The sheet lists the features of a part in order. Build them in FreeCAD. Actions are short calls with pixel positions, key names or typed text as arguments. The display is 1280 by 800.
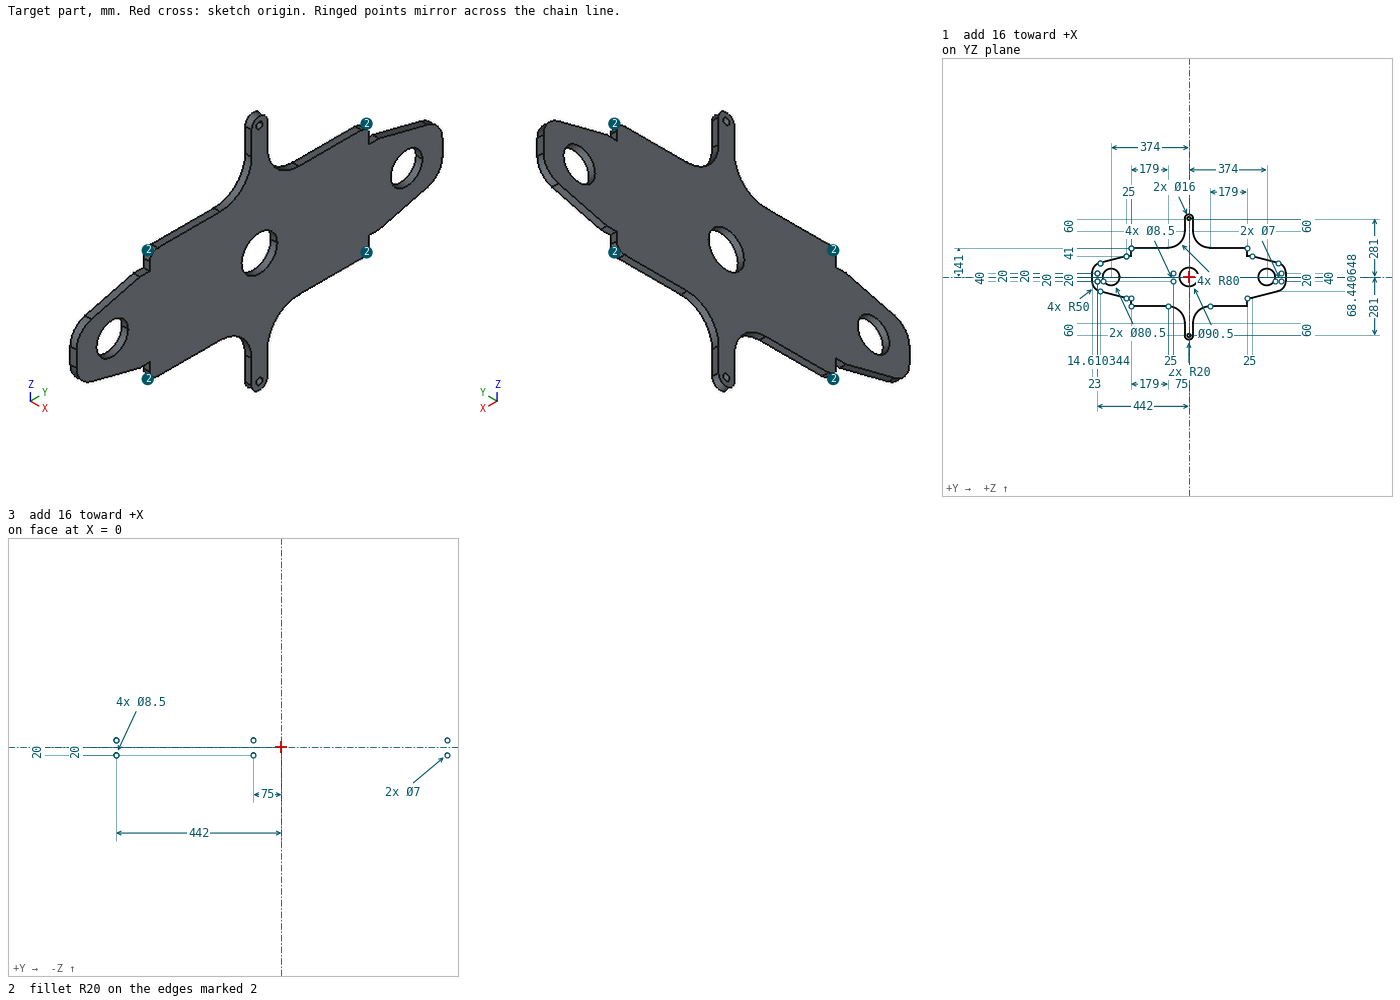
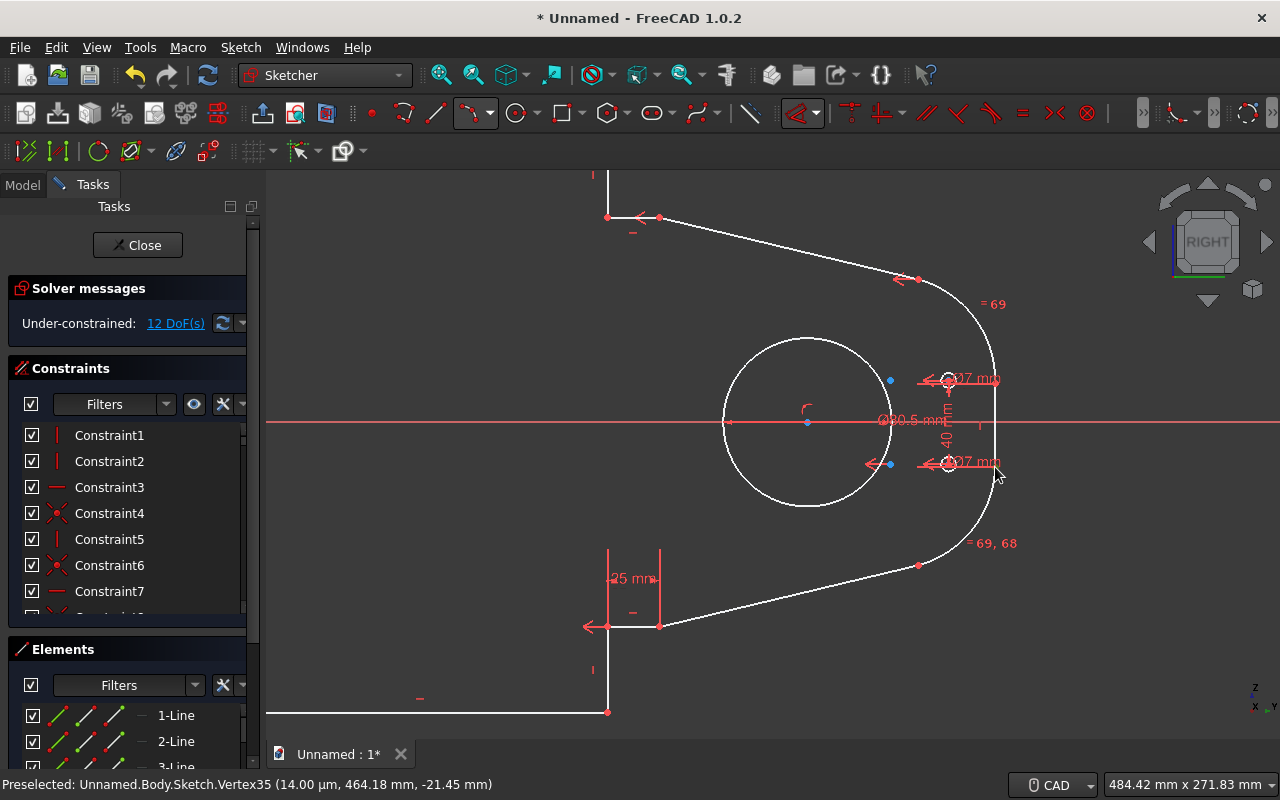
key(i)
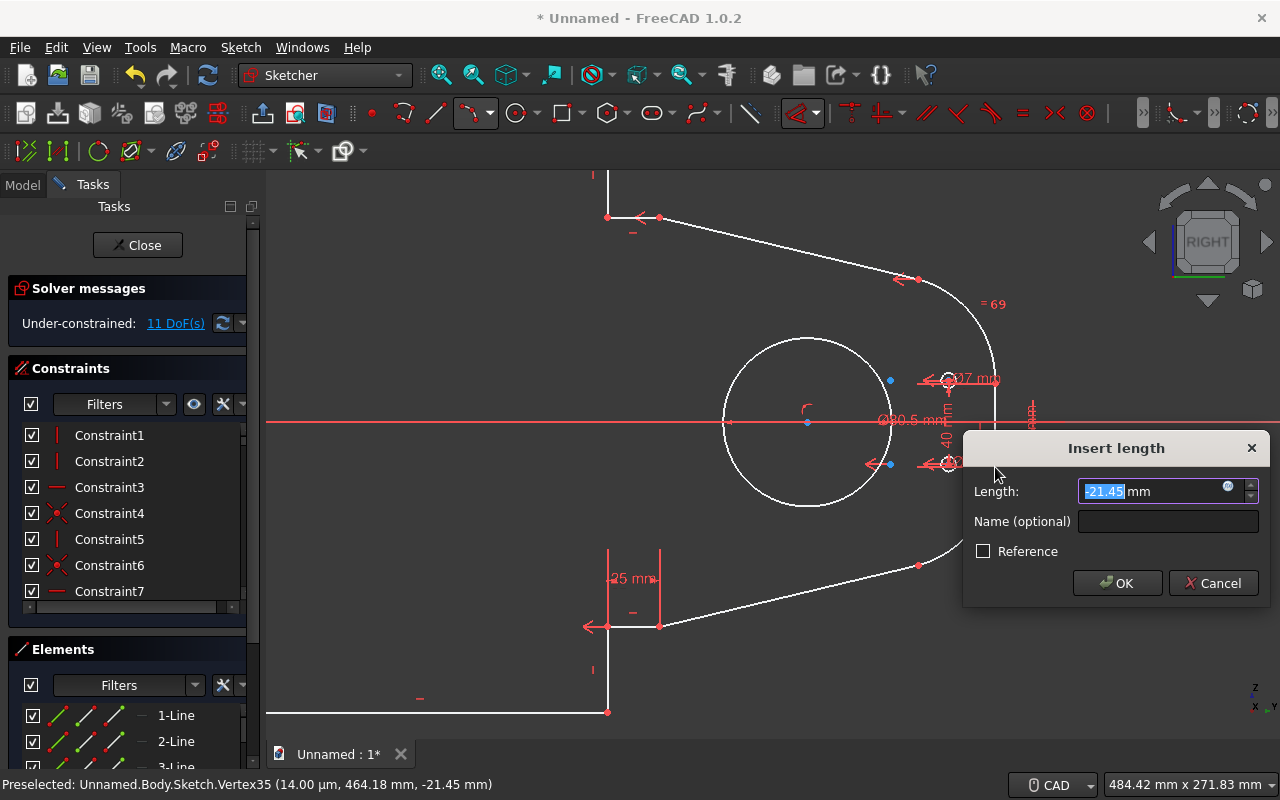
text(-20)
key(Return)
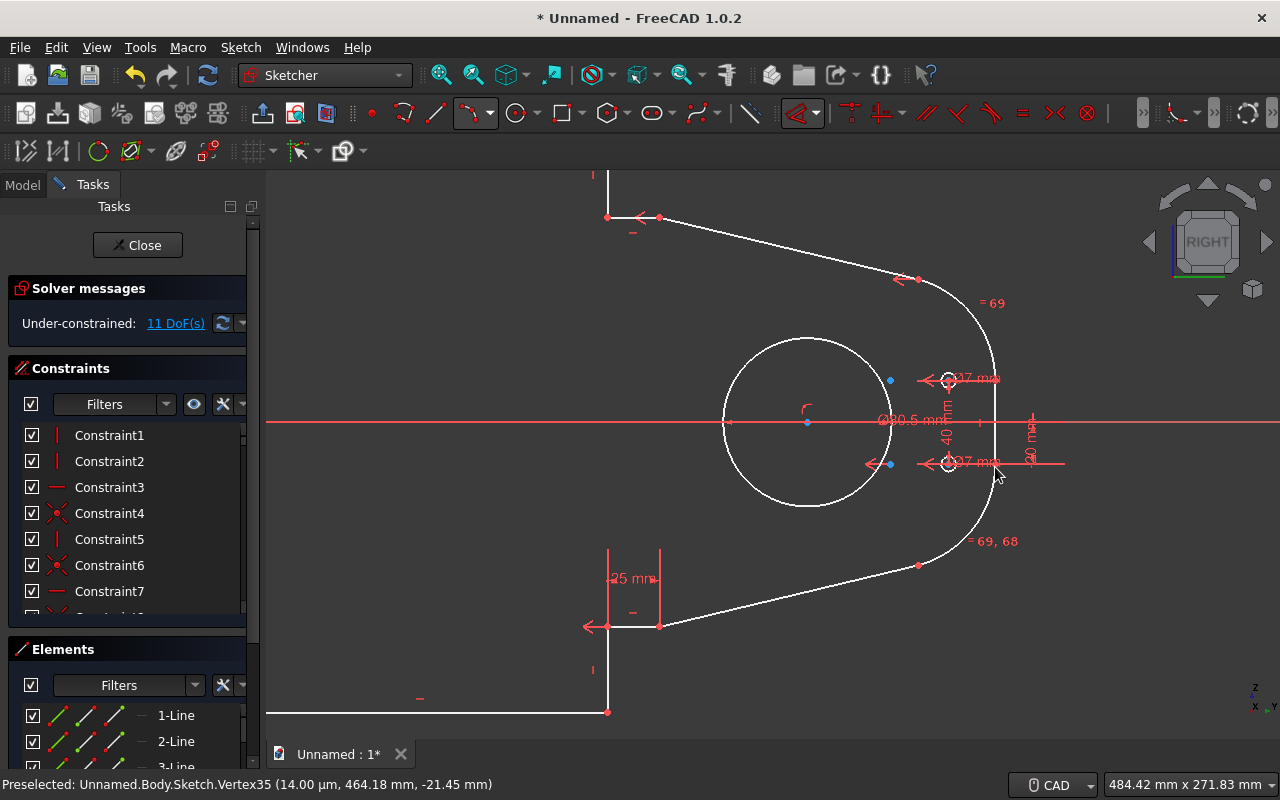
scroll(998, 468, down, 6)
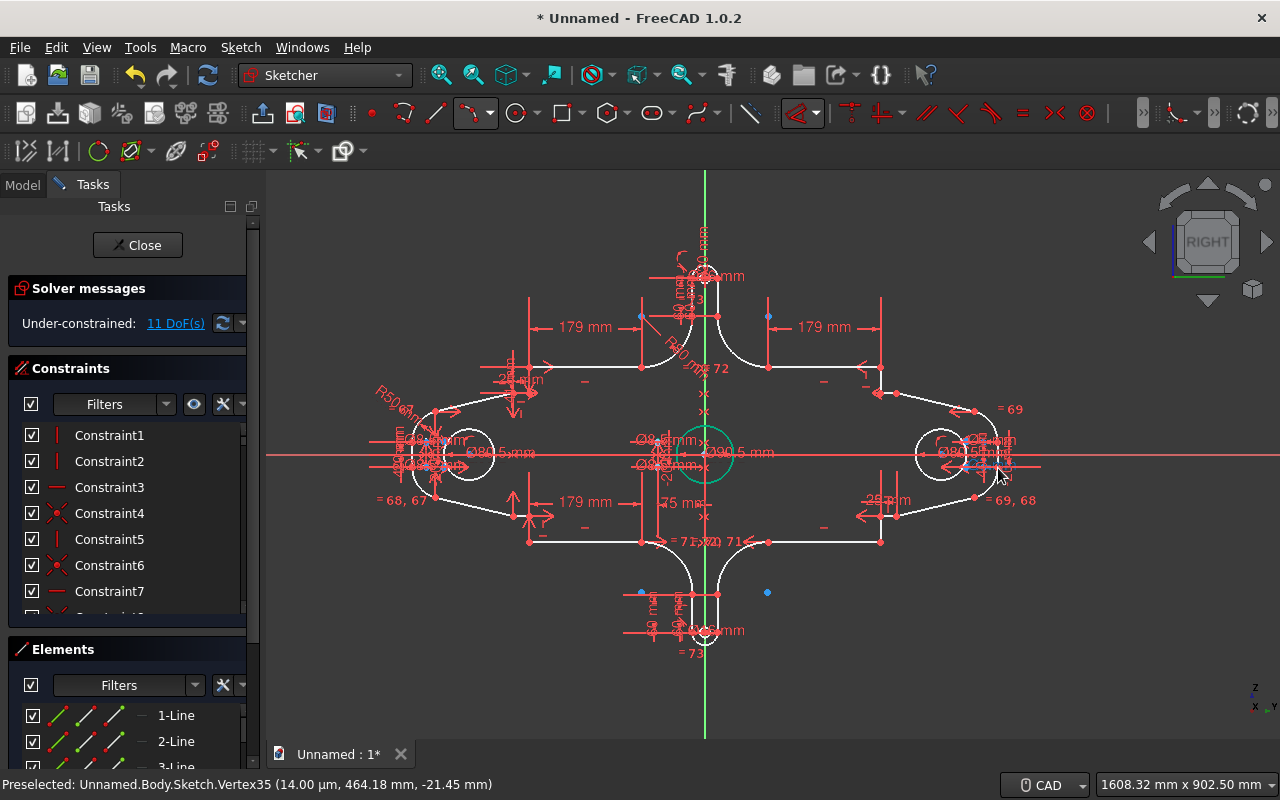
scroll(444, 442, up, 6)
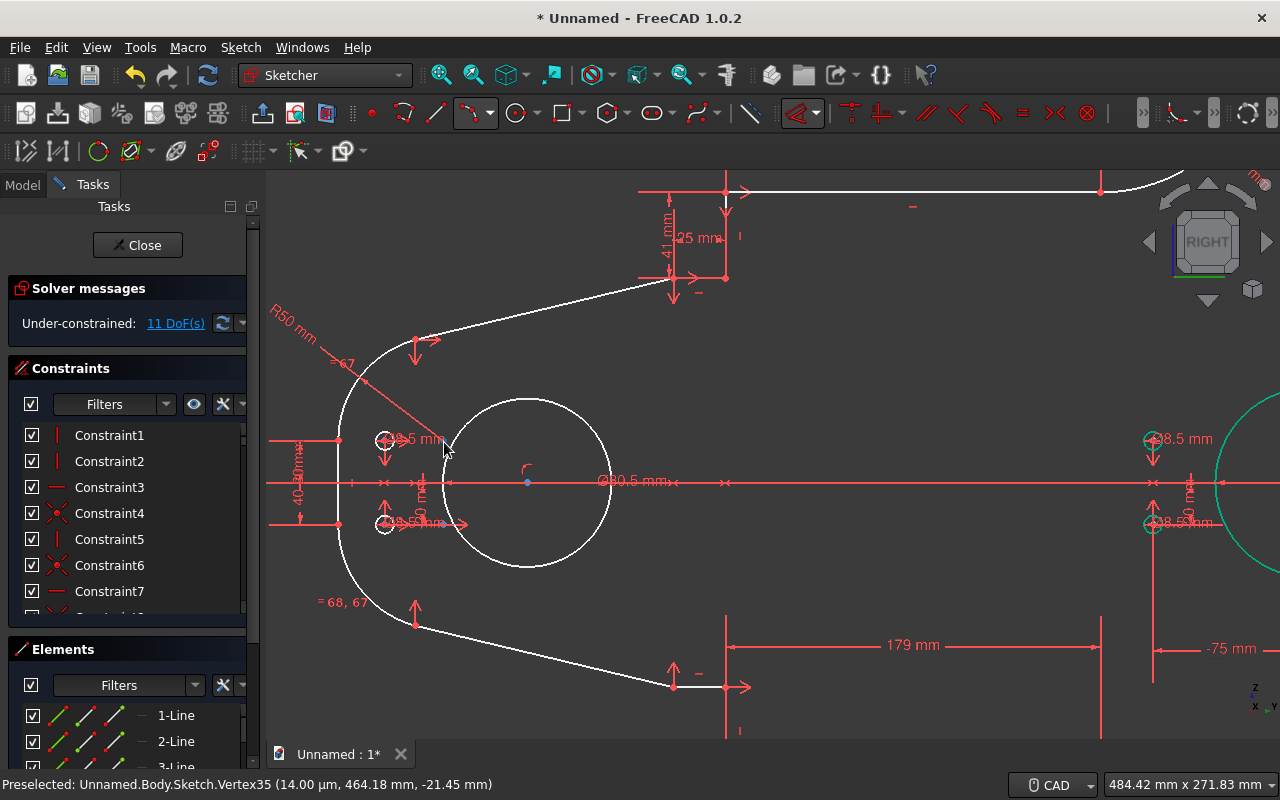
click(443, 441)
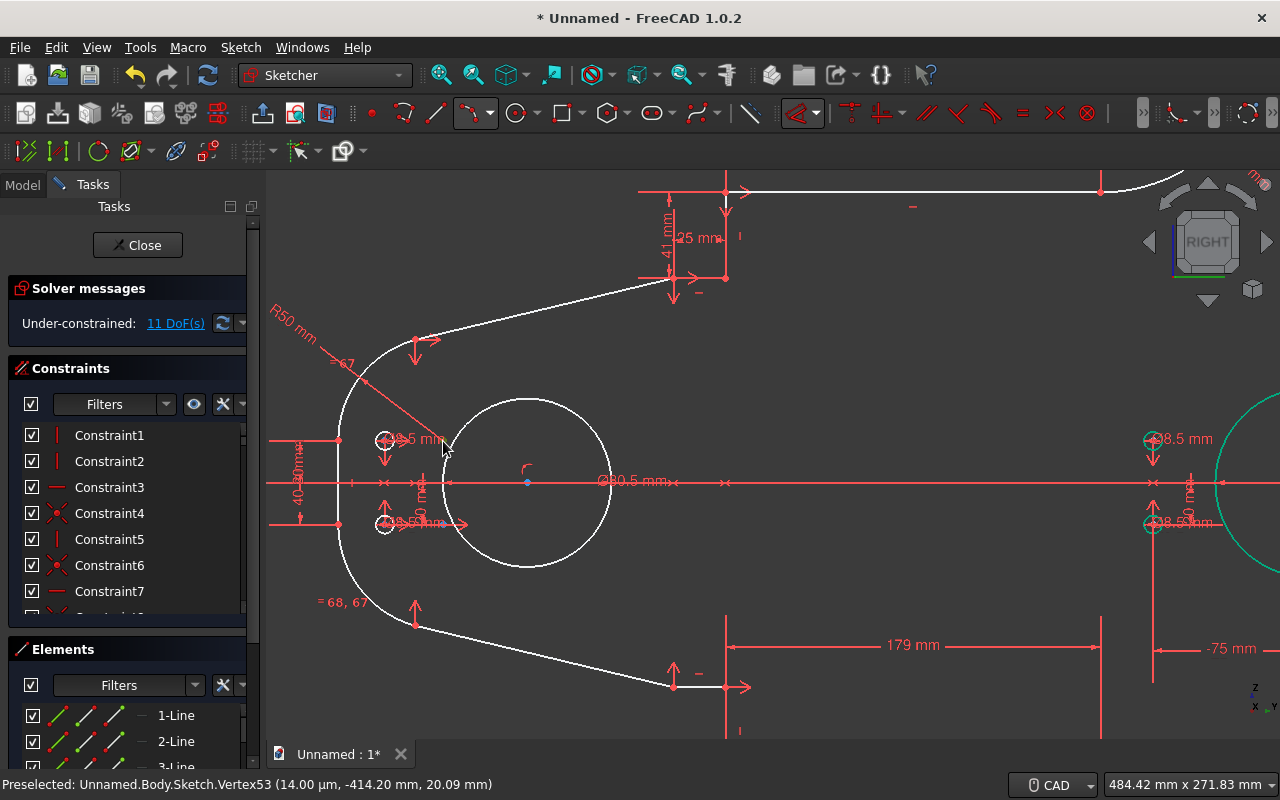
click(818, 114)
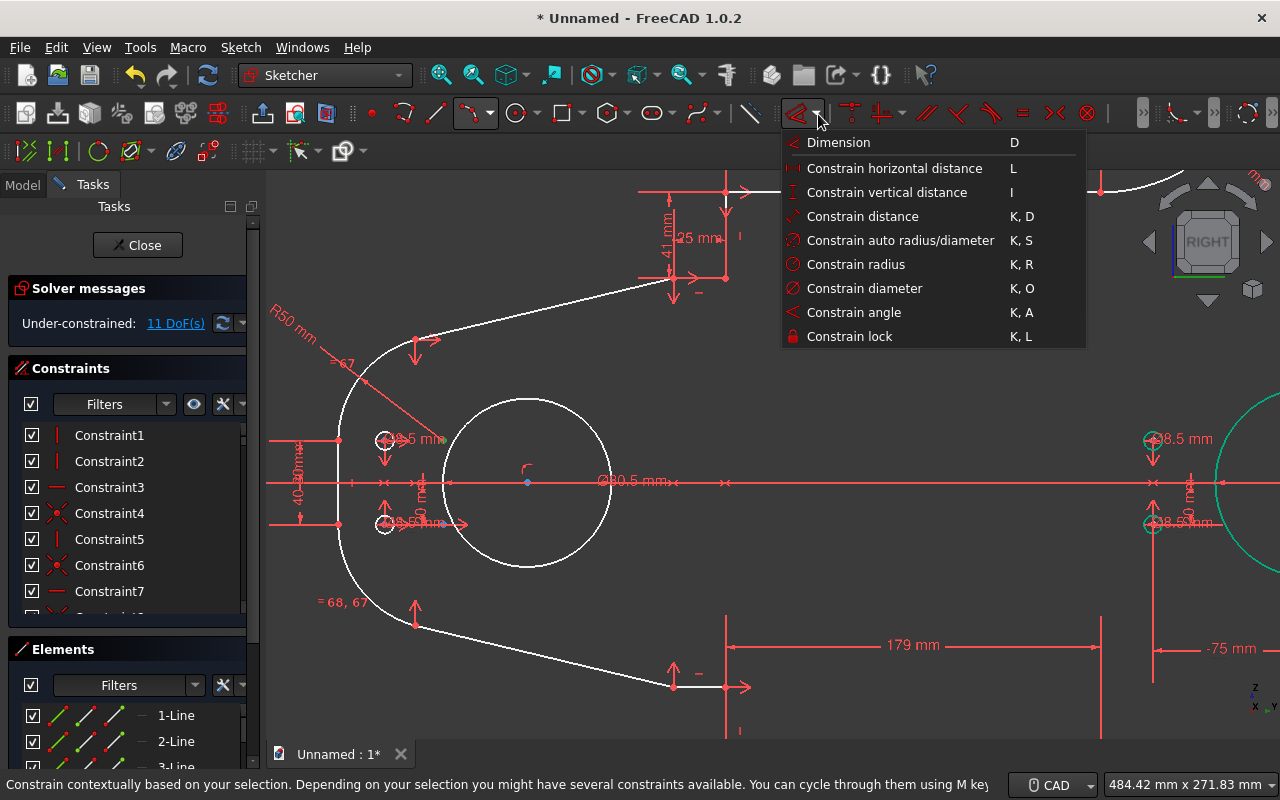
click(934, 192)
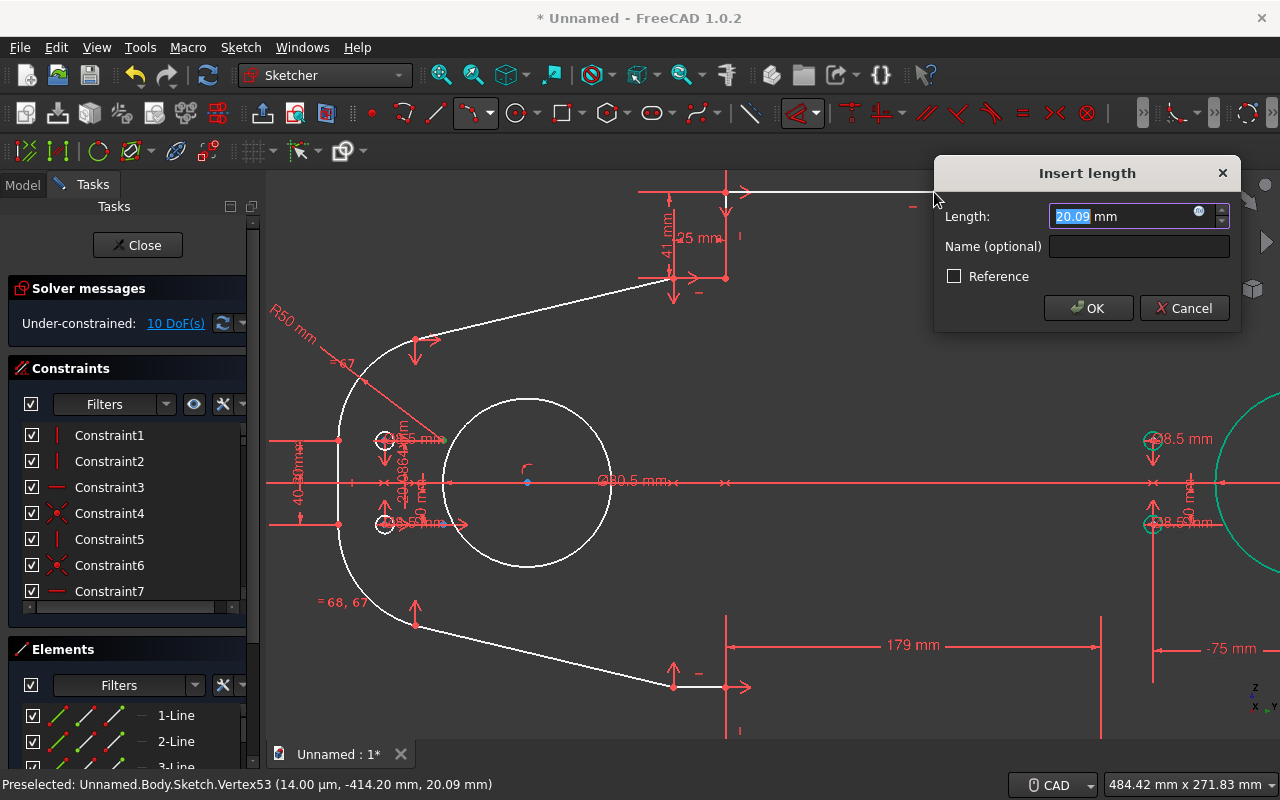
text(20)
key(Return)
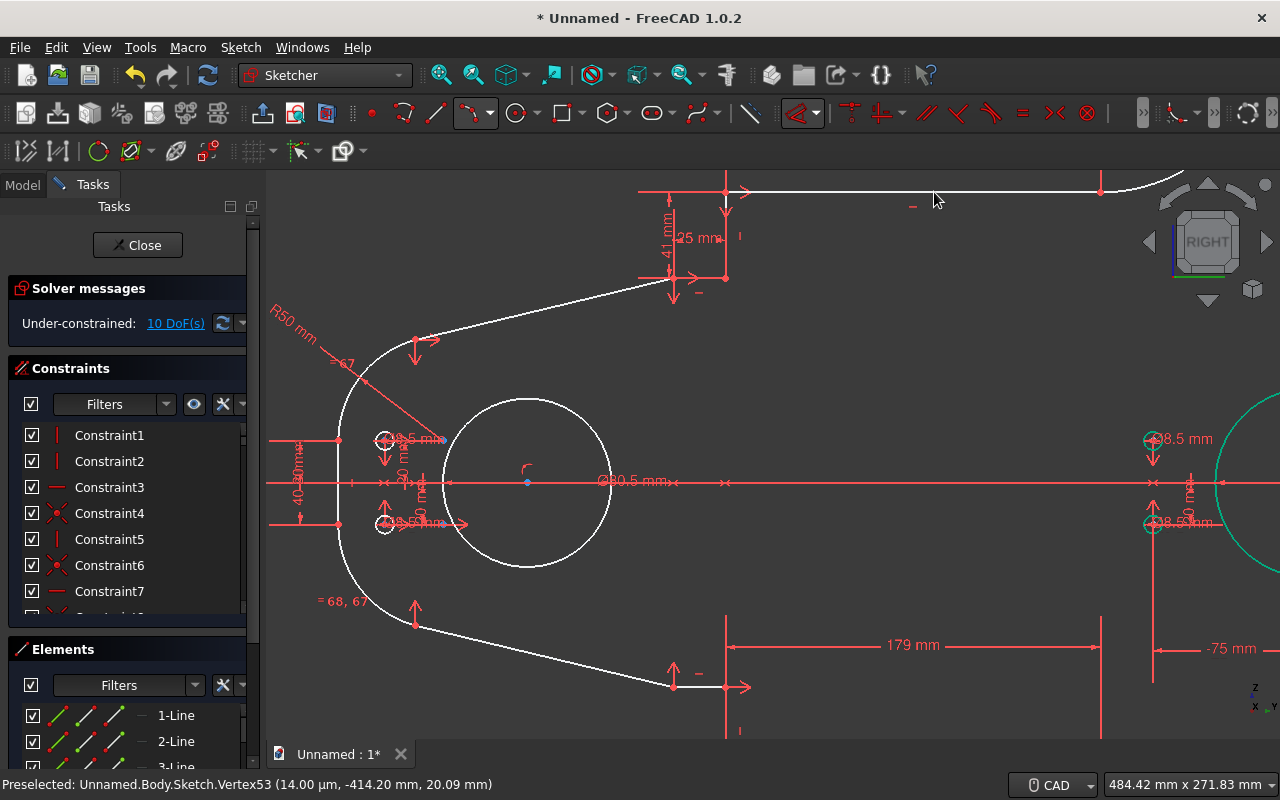
click(385, 525)